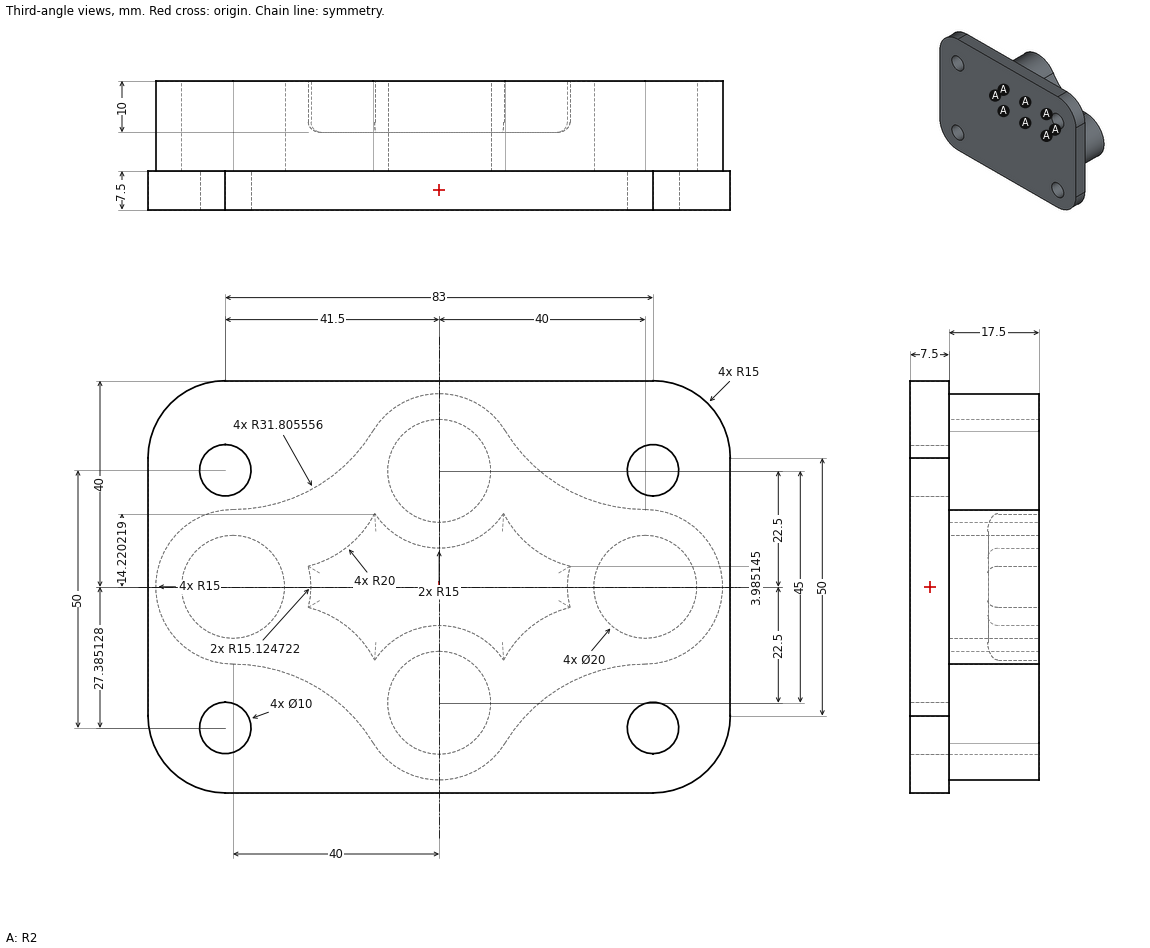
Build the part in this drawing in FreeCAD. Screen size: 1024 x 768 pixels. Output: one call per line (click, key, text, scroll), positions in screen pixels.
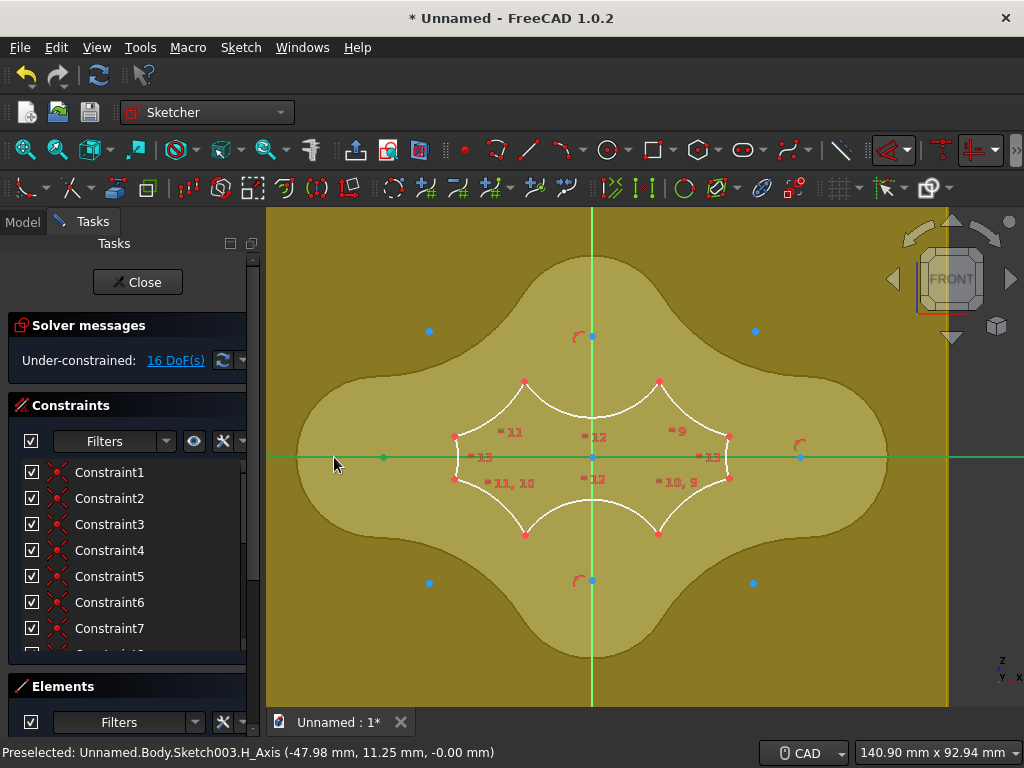
click(942, 150)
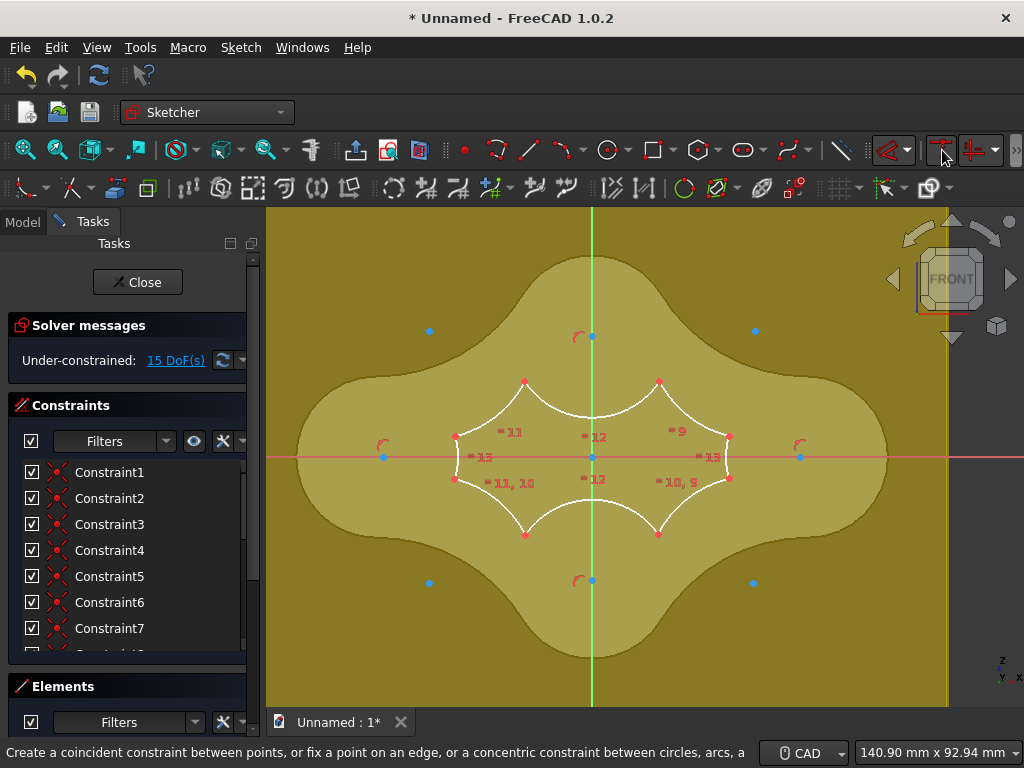
click(755, 331)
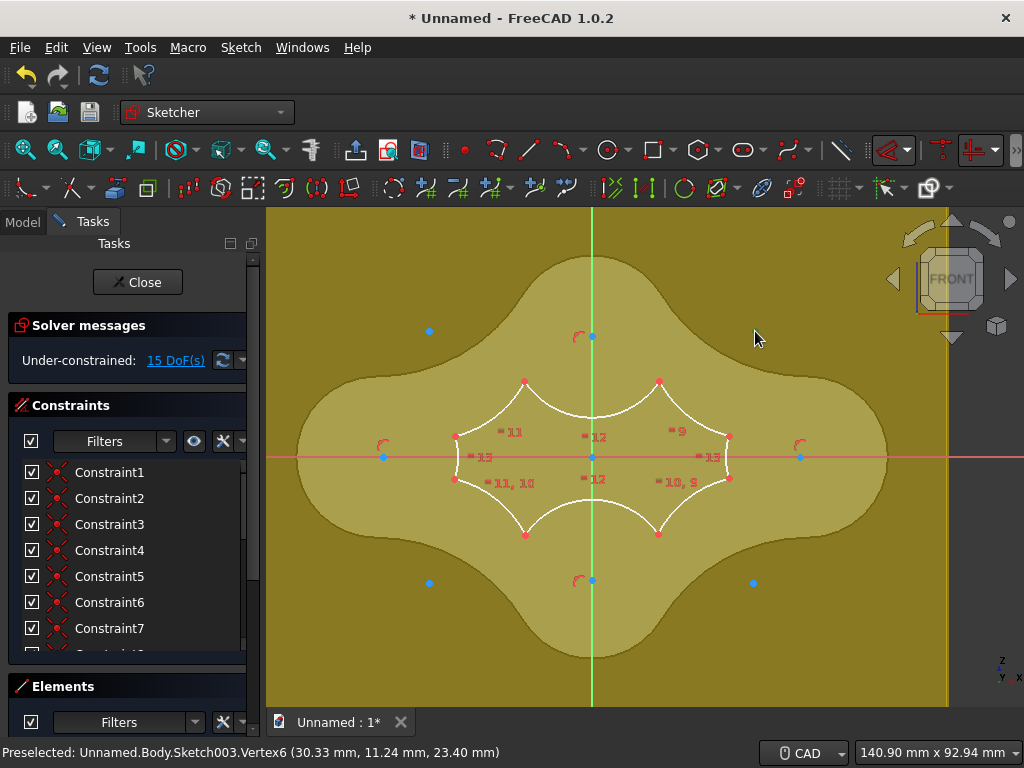
click(754, 584)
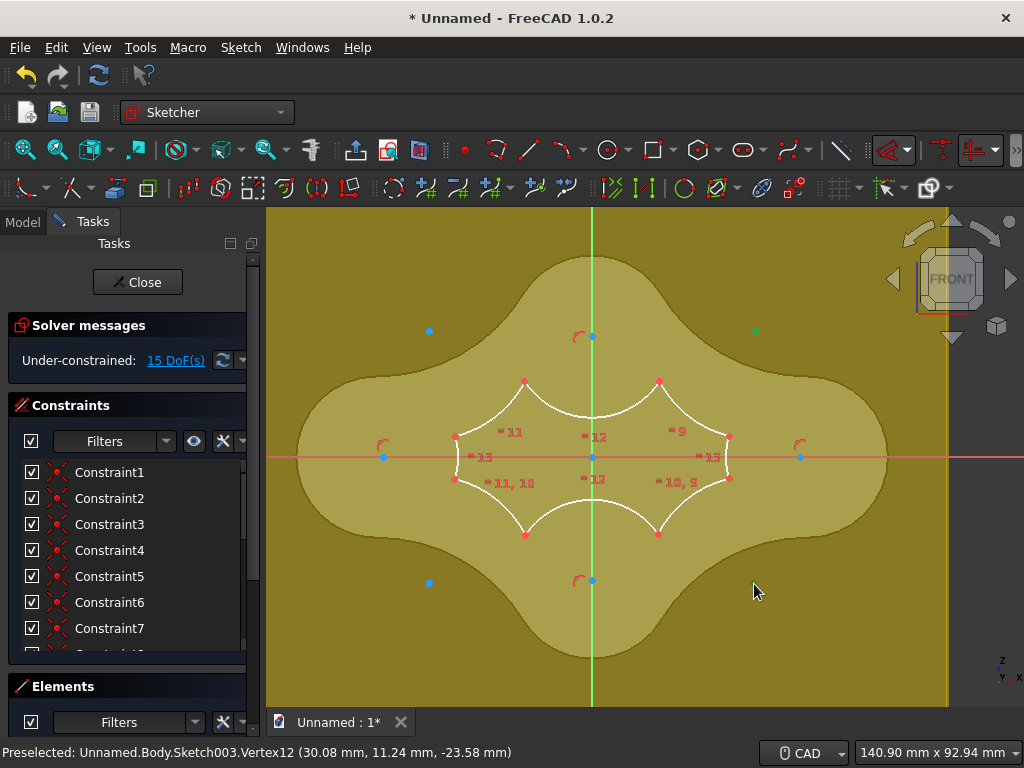
click(334, 457)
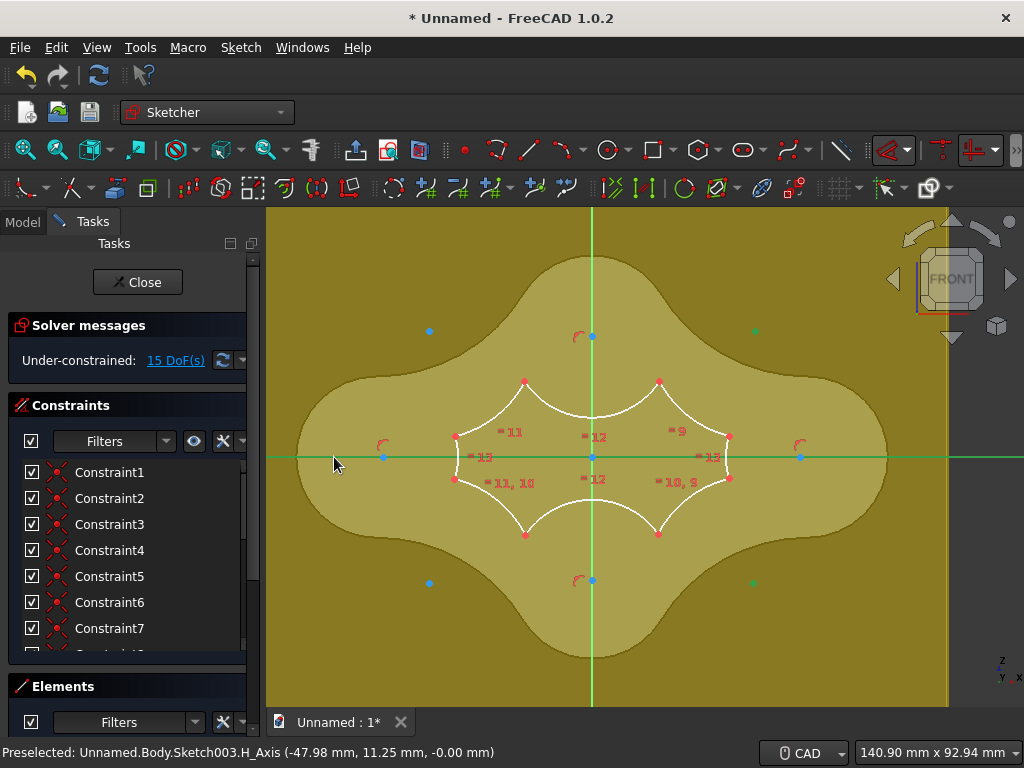
key(s)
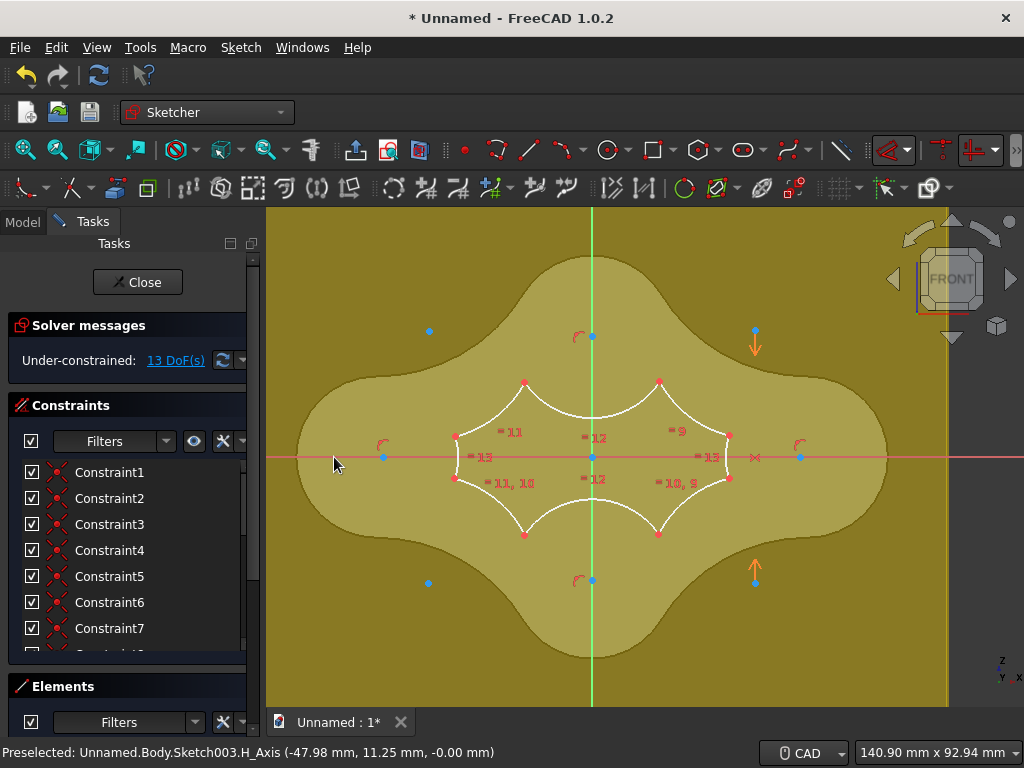
click(755, 584)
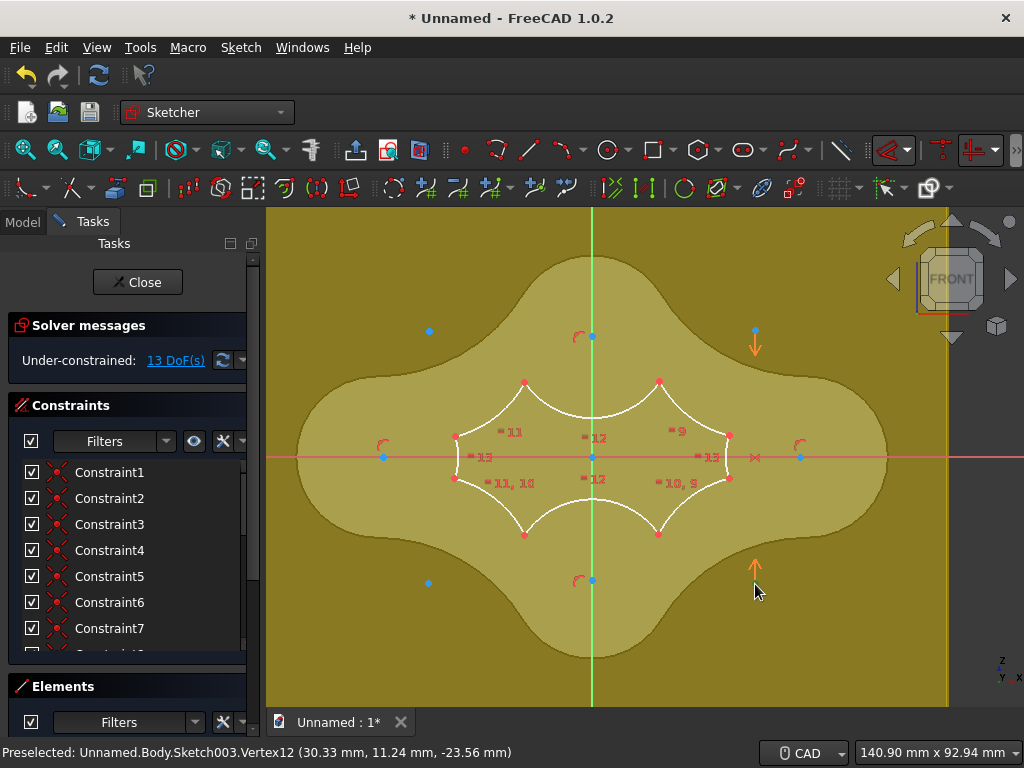
click(428, 584)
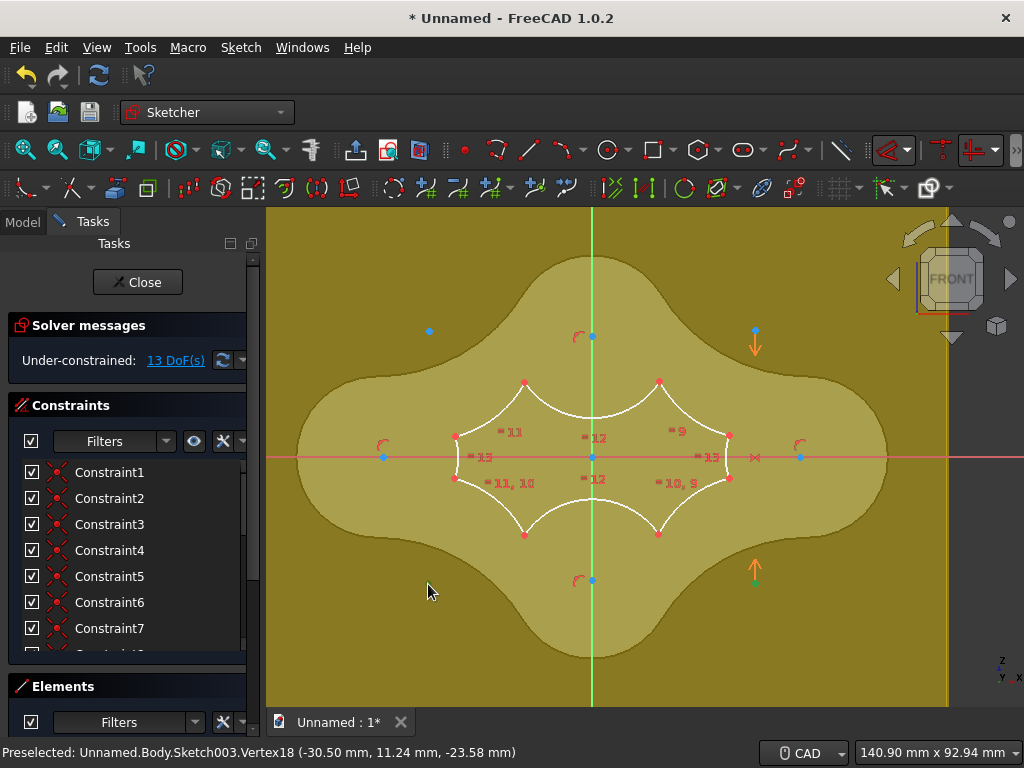
click(592, 647)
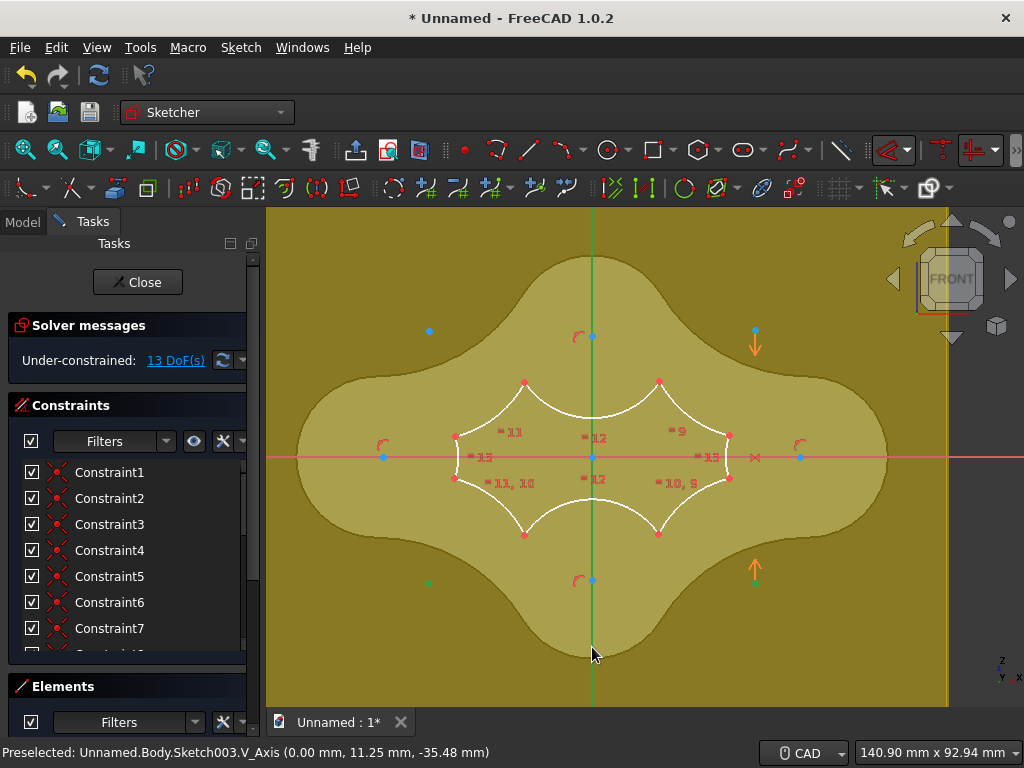
key(s)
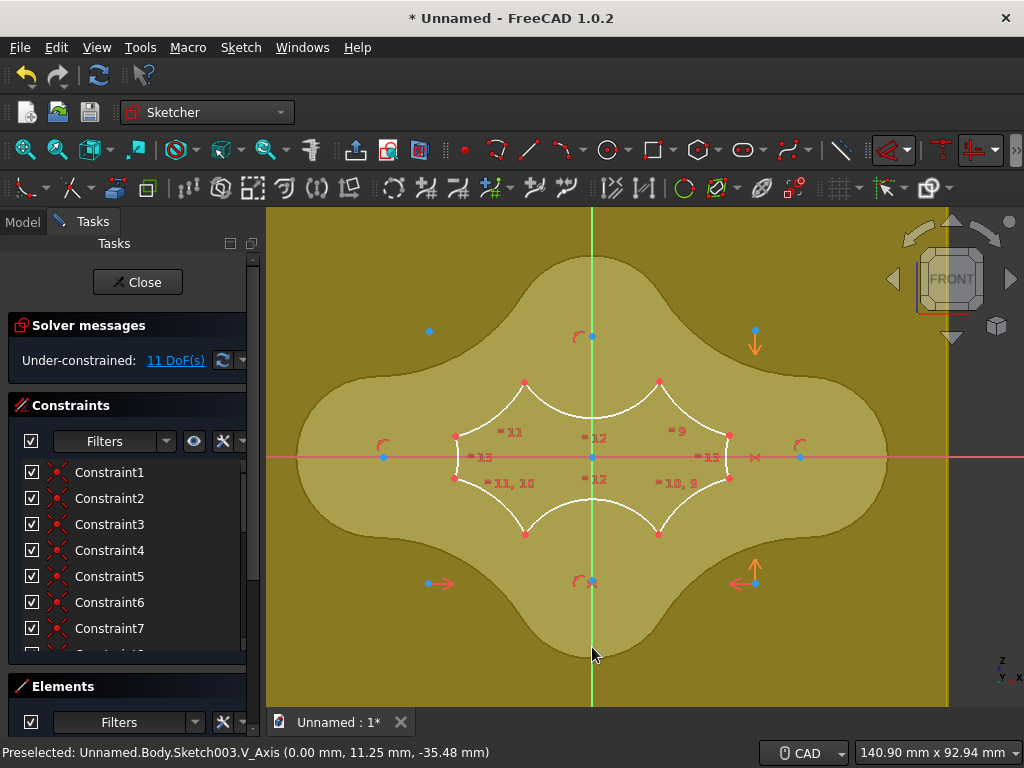
click(755, 330)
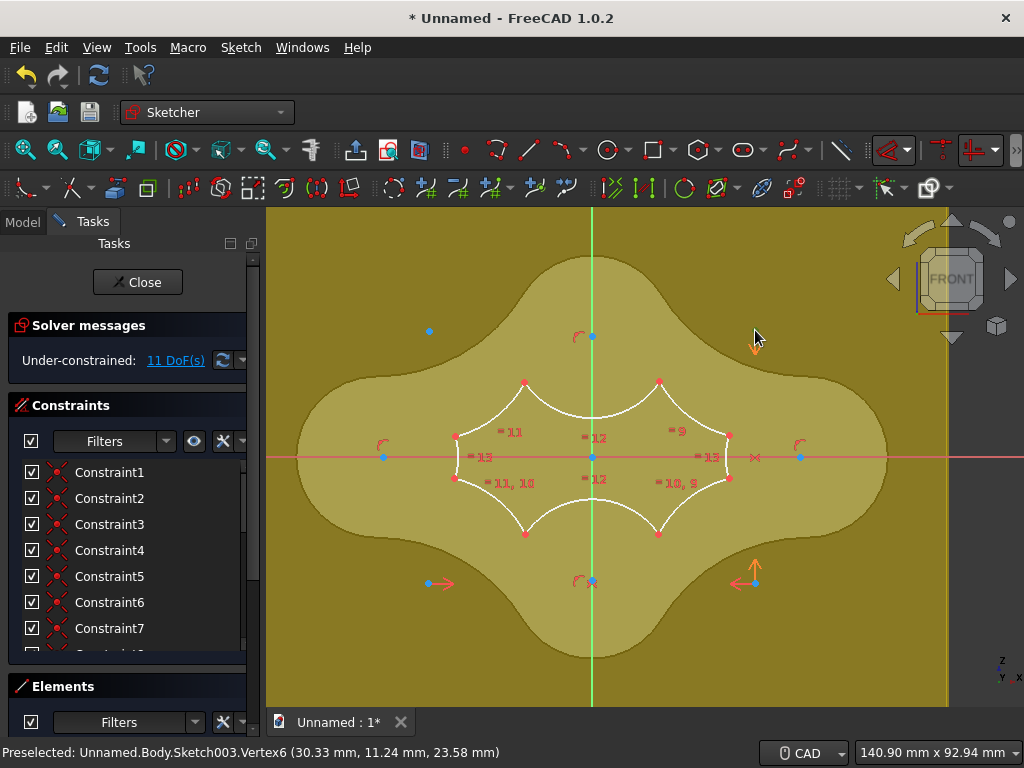
click(429, 331)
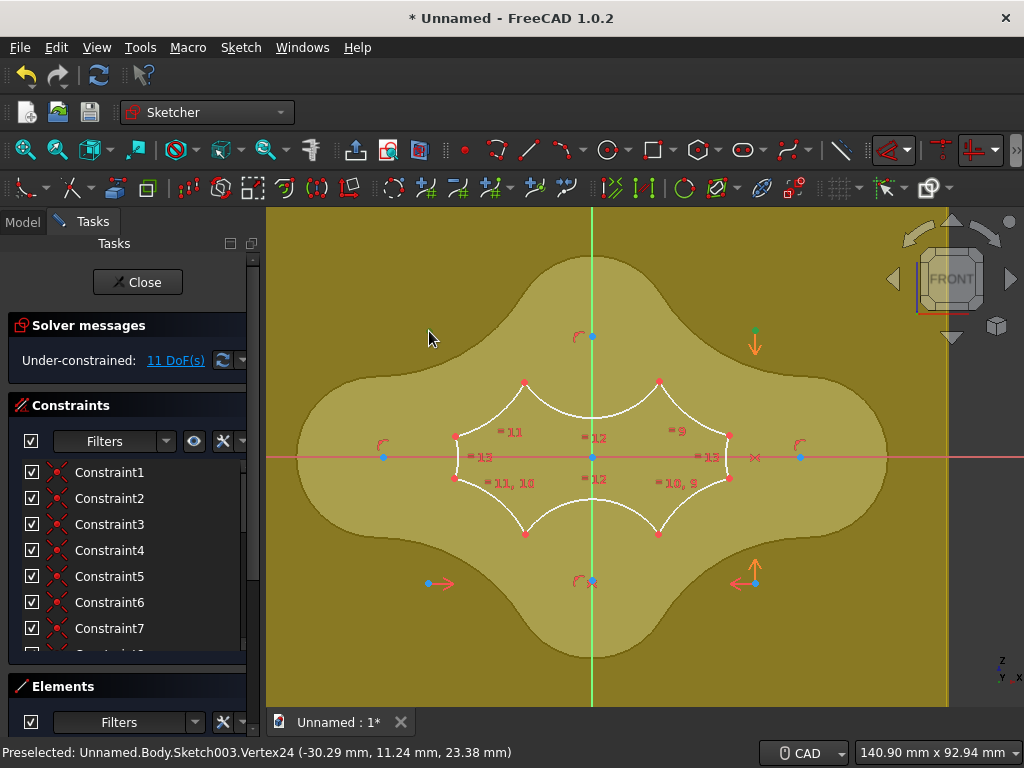
click(592, 647)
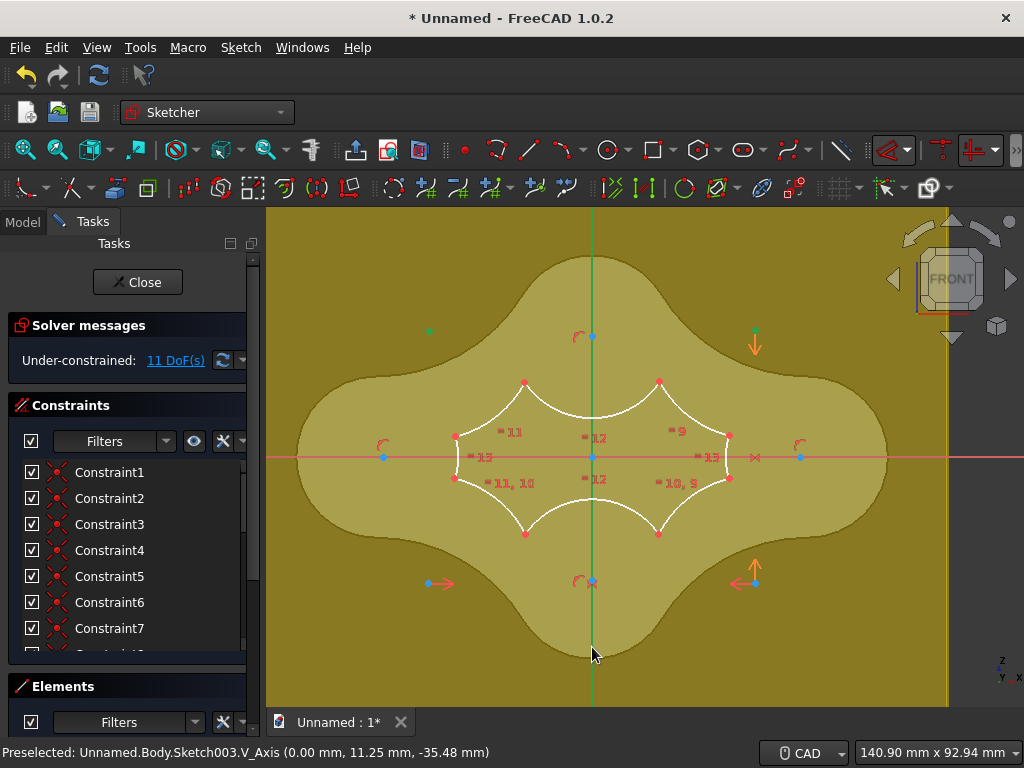
key(s)